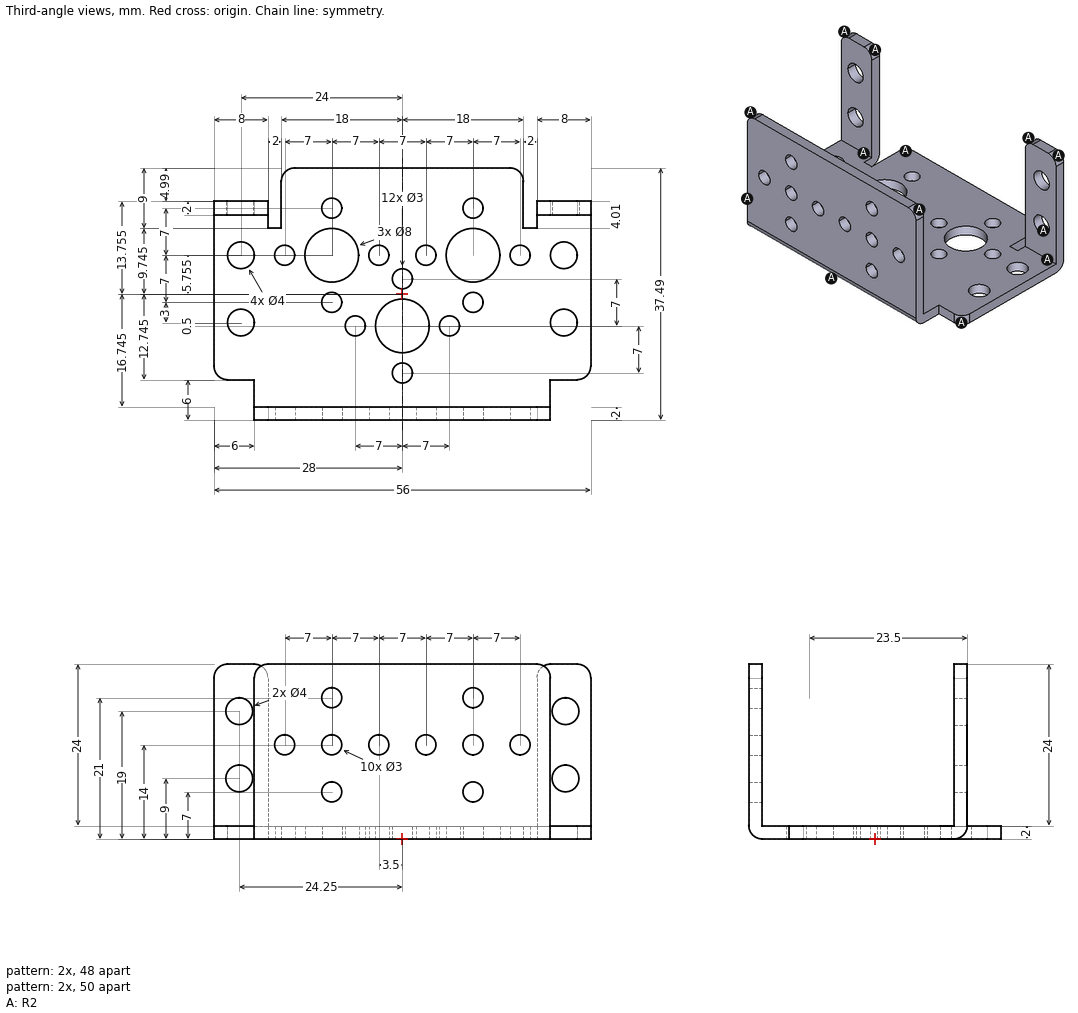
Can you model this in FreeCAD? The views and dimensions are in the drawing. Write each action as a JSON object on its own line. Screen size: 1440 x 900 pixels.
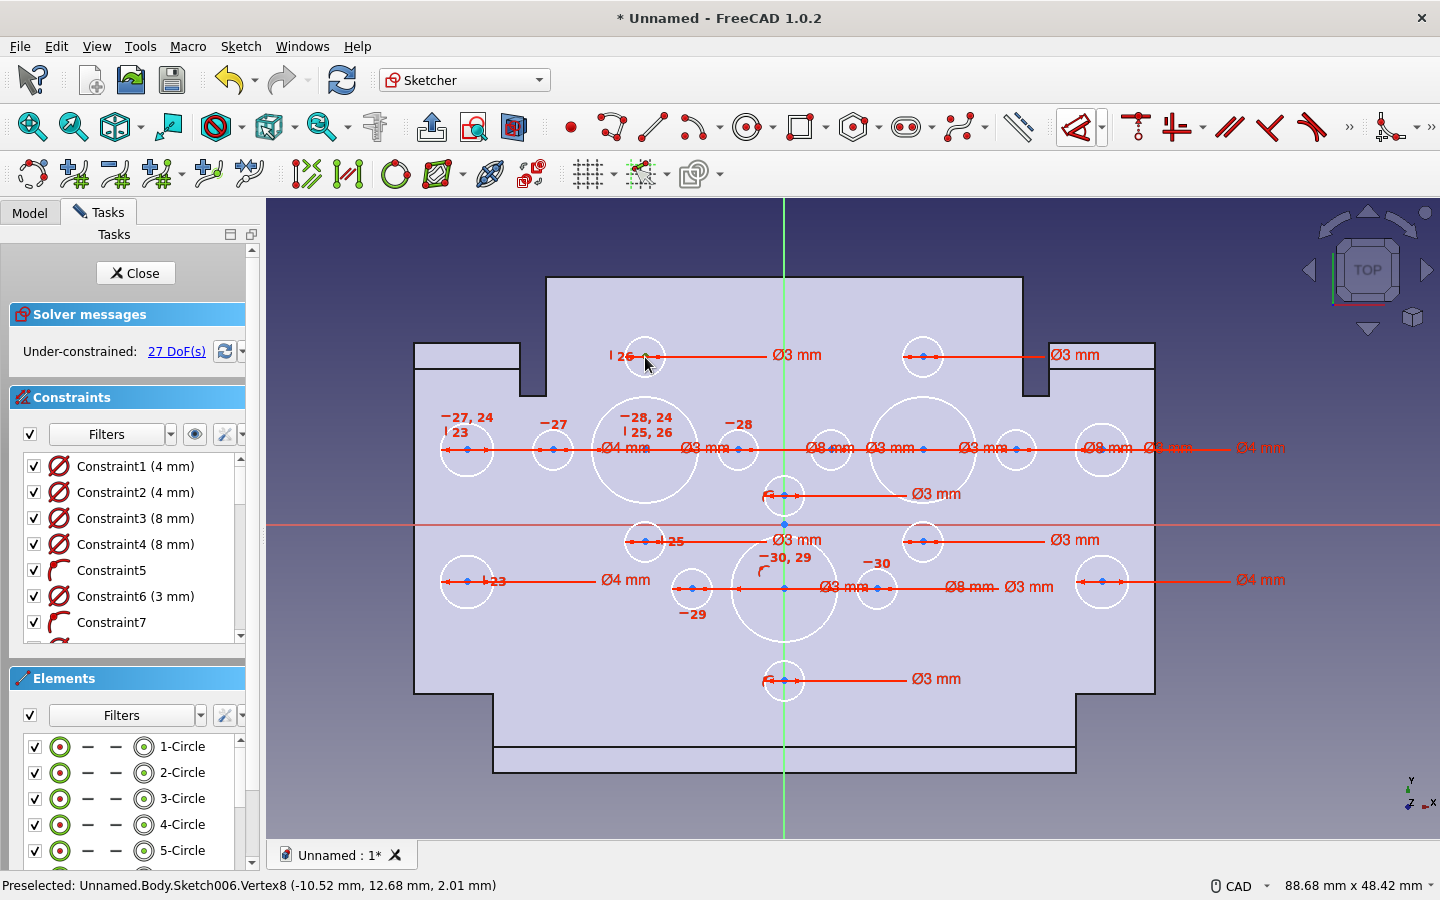
{"action": "left_click", "coordinate": [923, 357]}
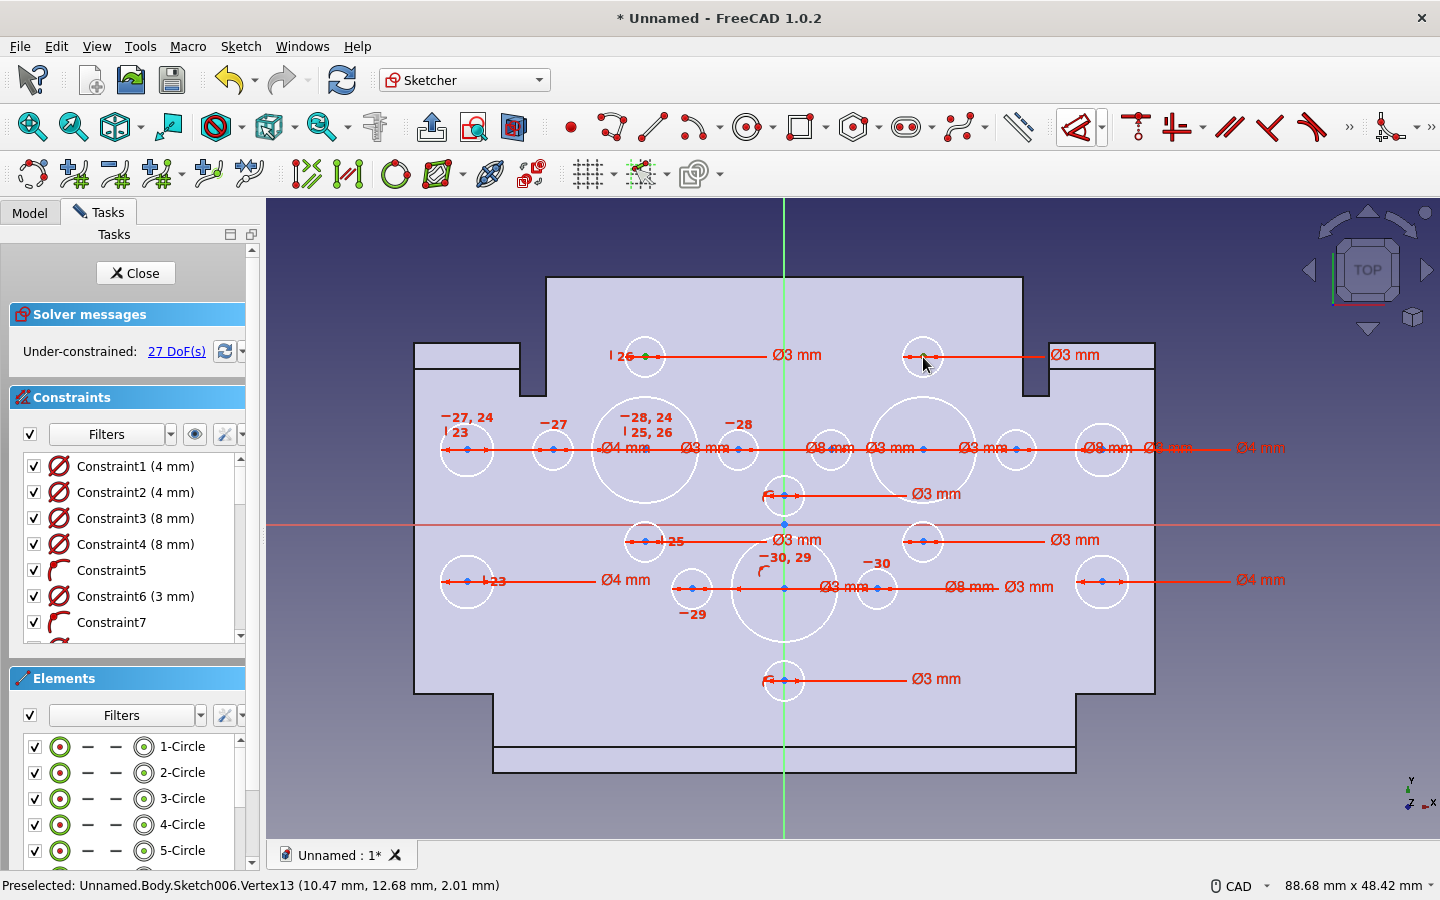
{"action": "key", "text": "h"}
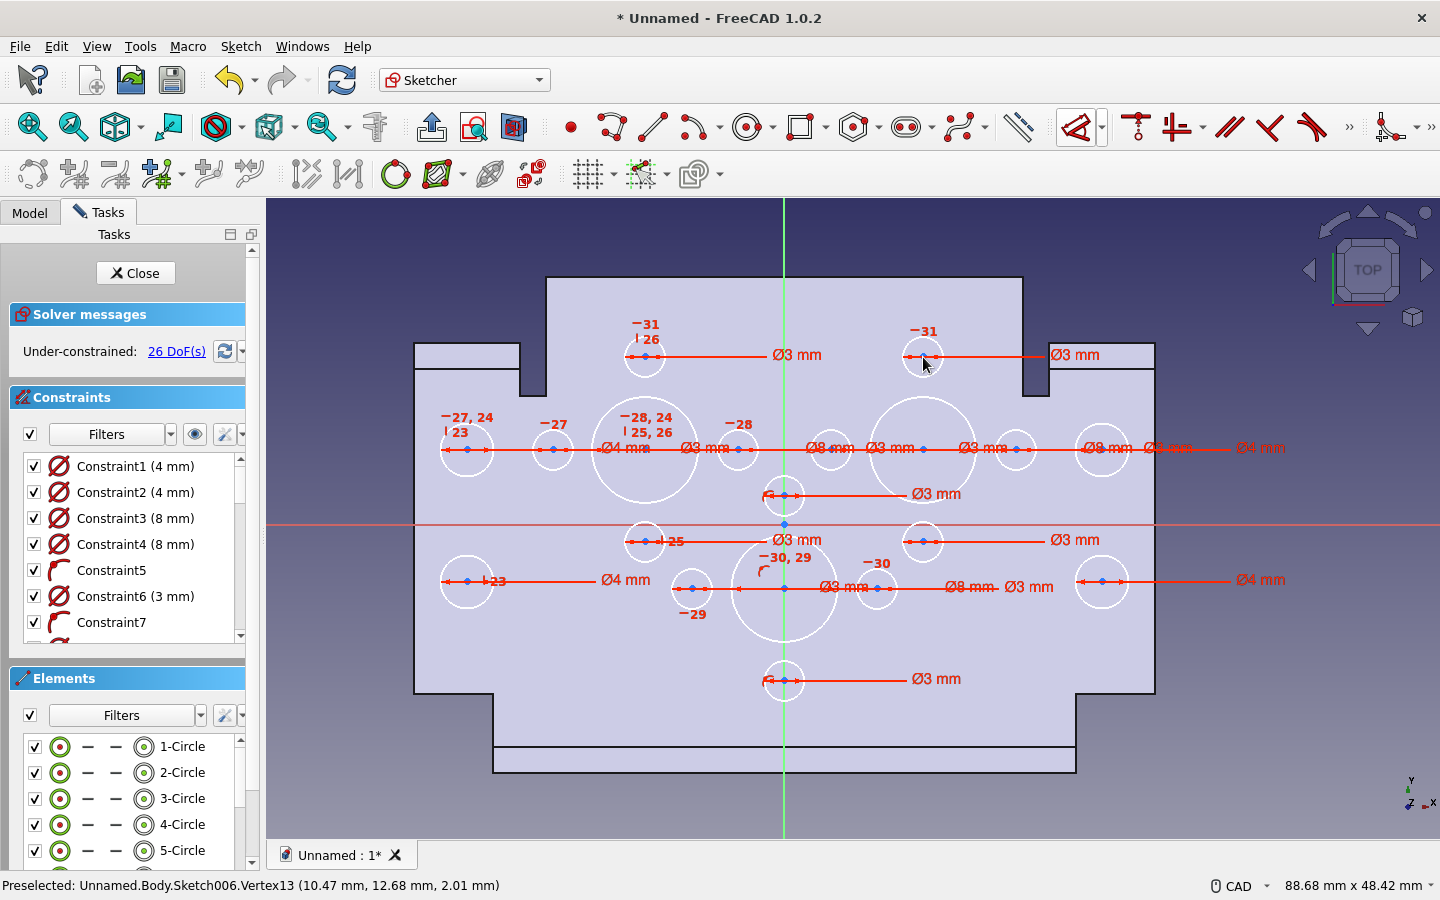
{"action": "left_click", "coordinate": [738, 450]}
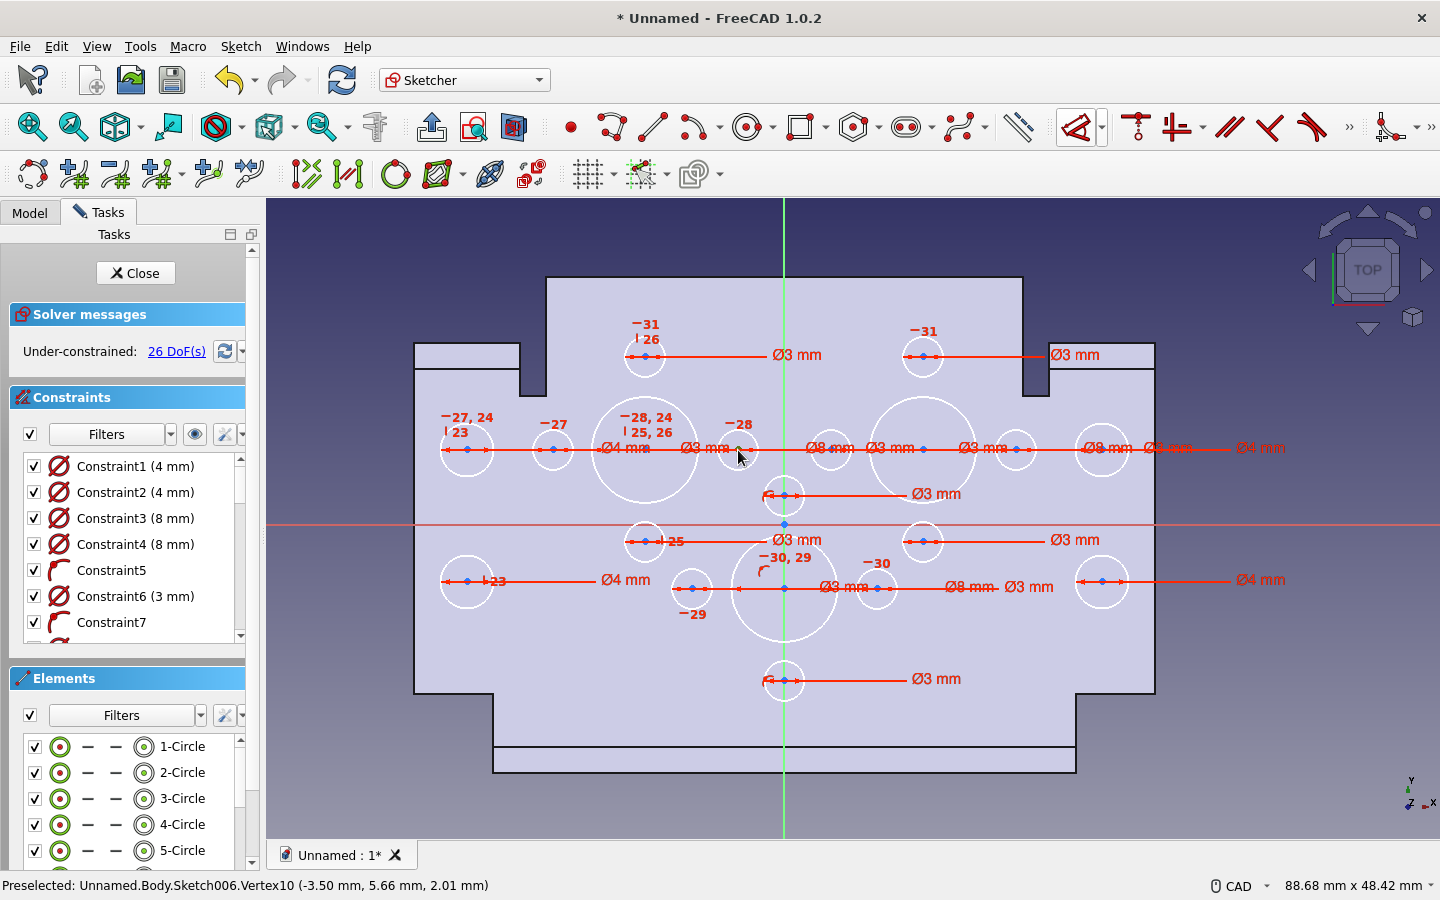
{"action": "left_click", "coordinate": [831, 450]}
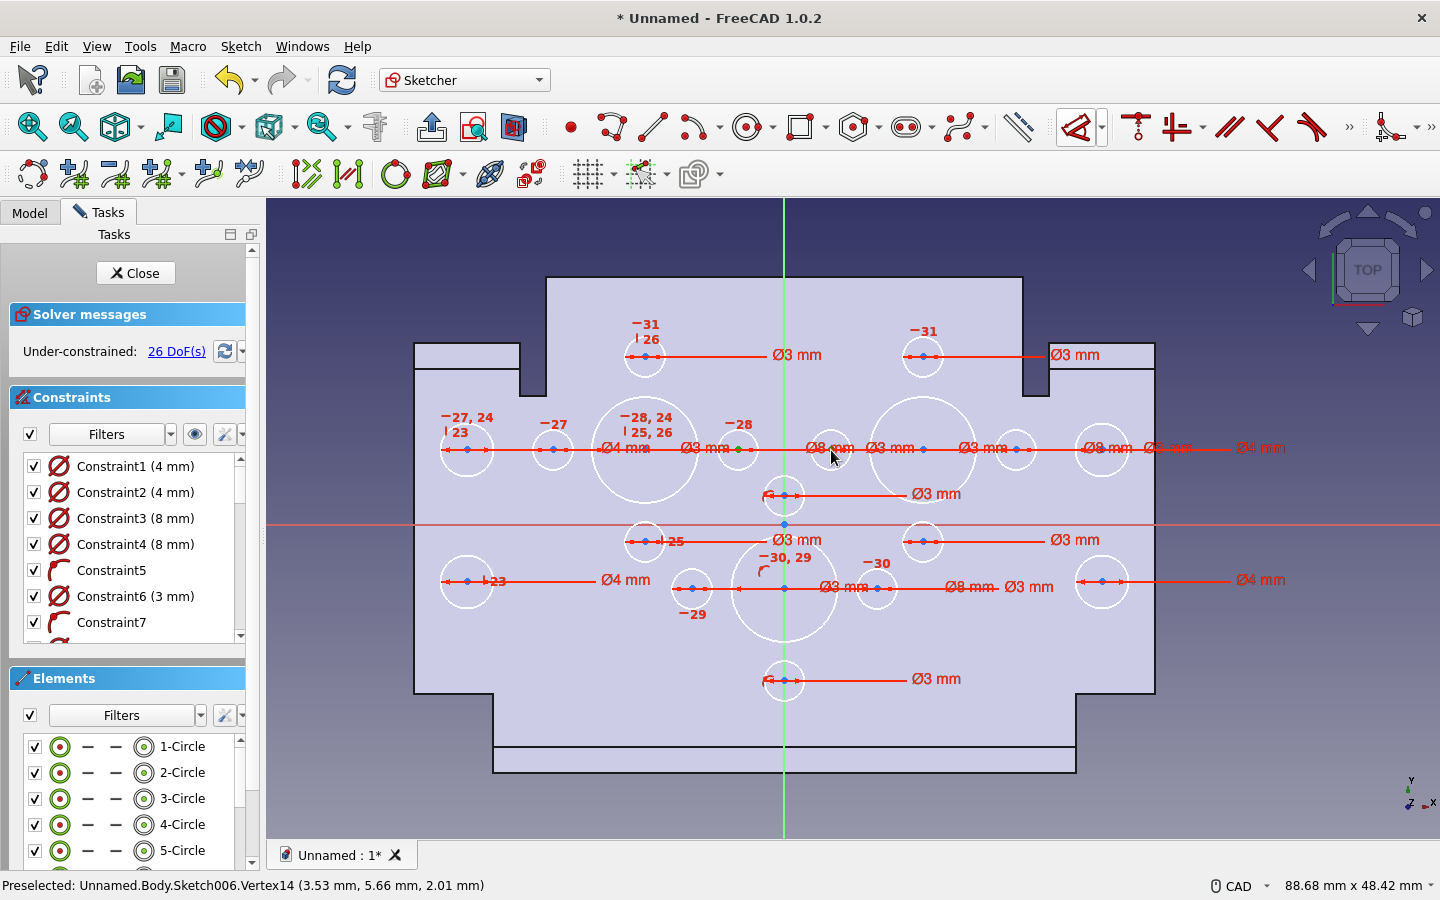
{"action": "key", "text": "h"}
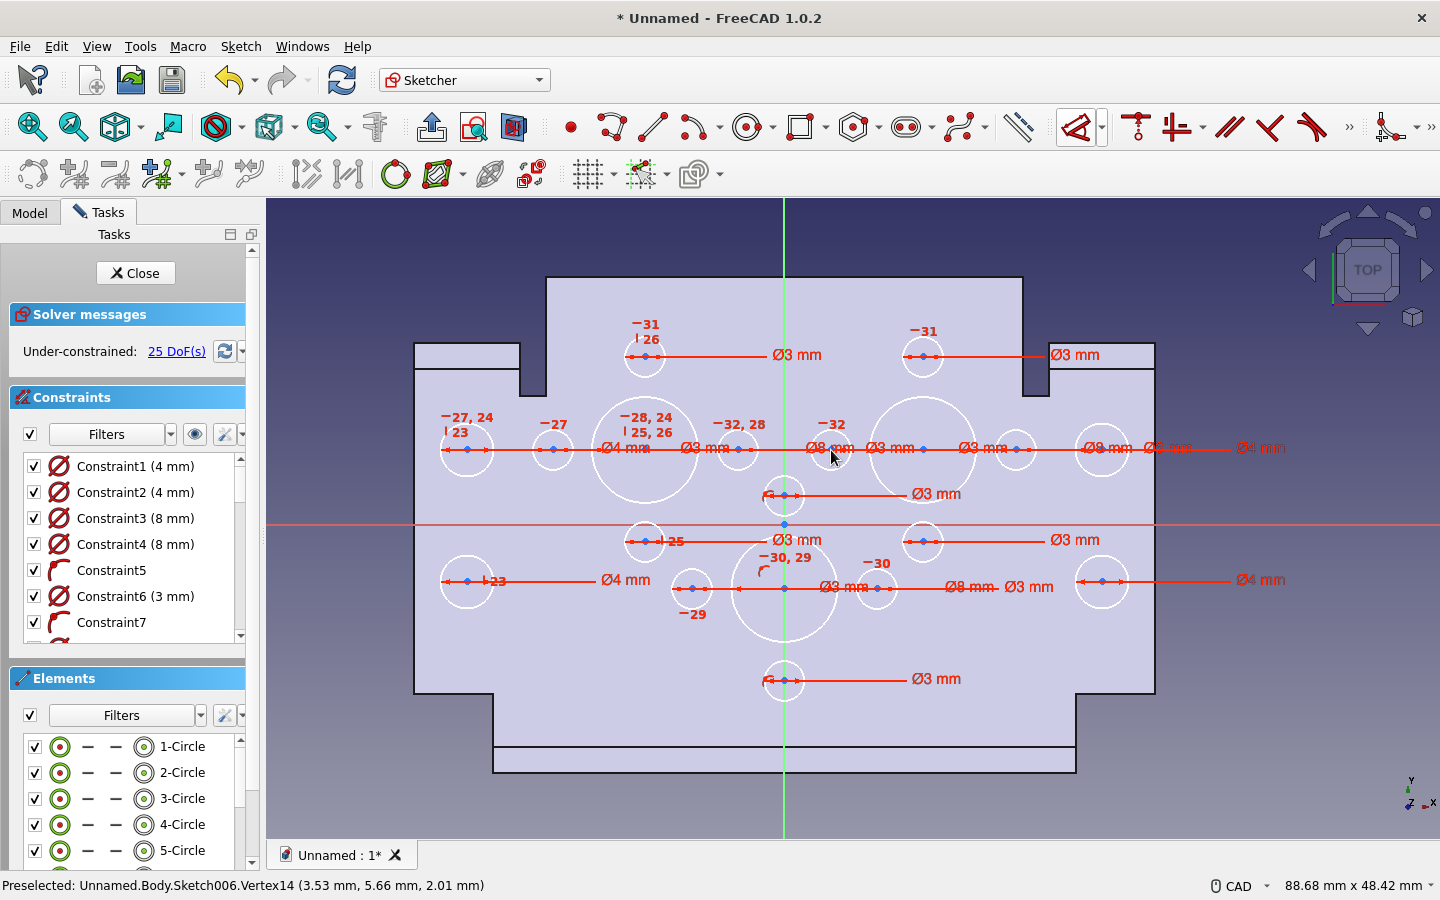
{"action": "left_click", "coordinate": [923, 357]}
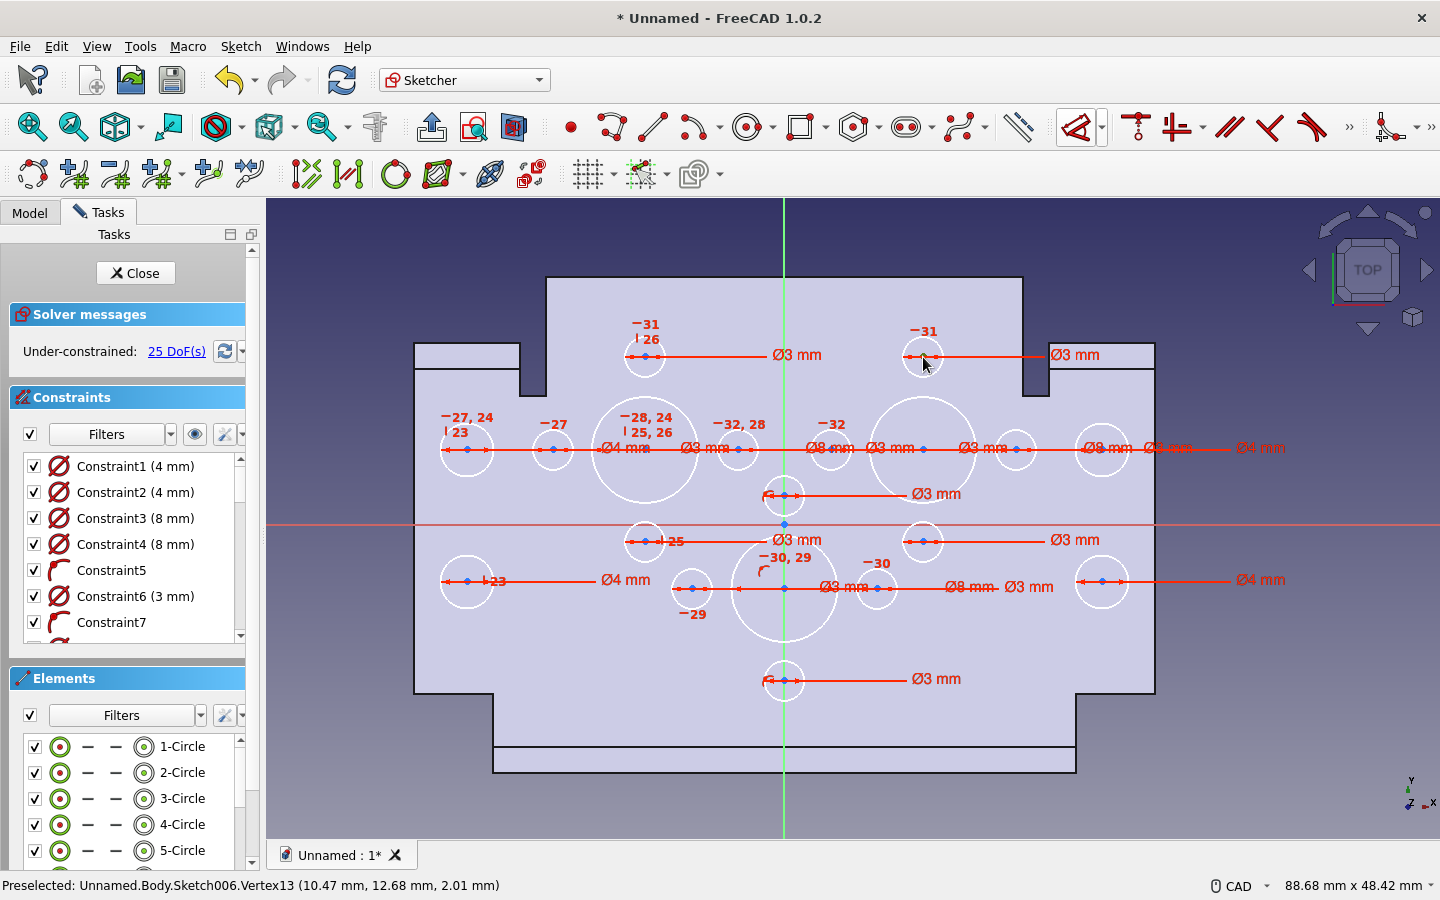
{"action": "left_click", "coordinate": [923, 542]}